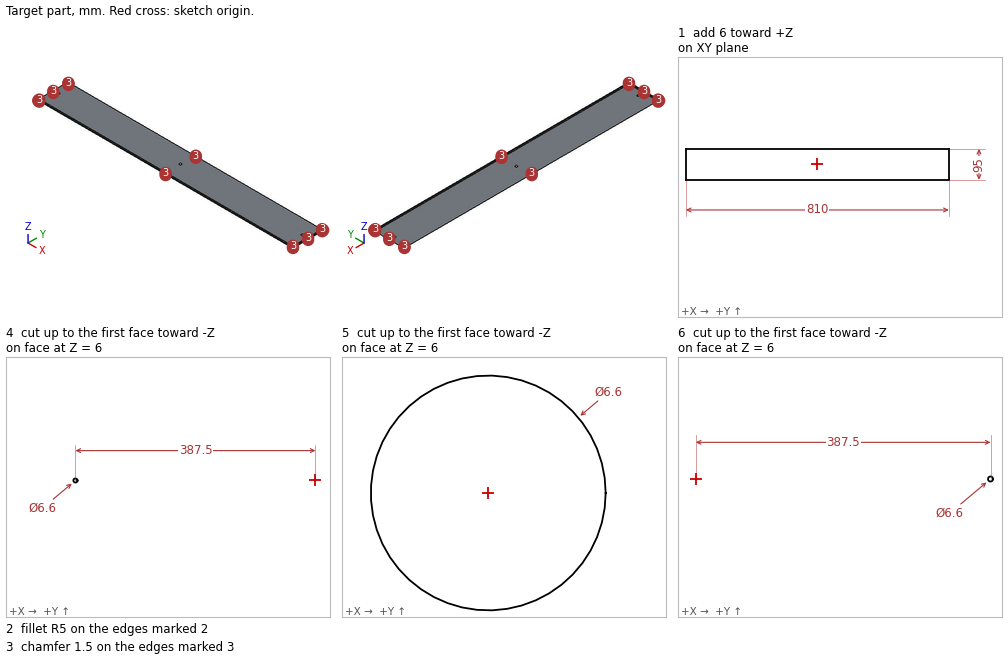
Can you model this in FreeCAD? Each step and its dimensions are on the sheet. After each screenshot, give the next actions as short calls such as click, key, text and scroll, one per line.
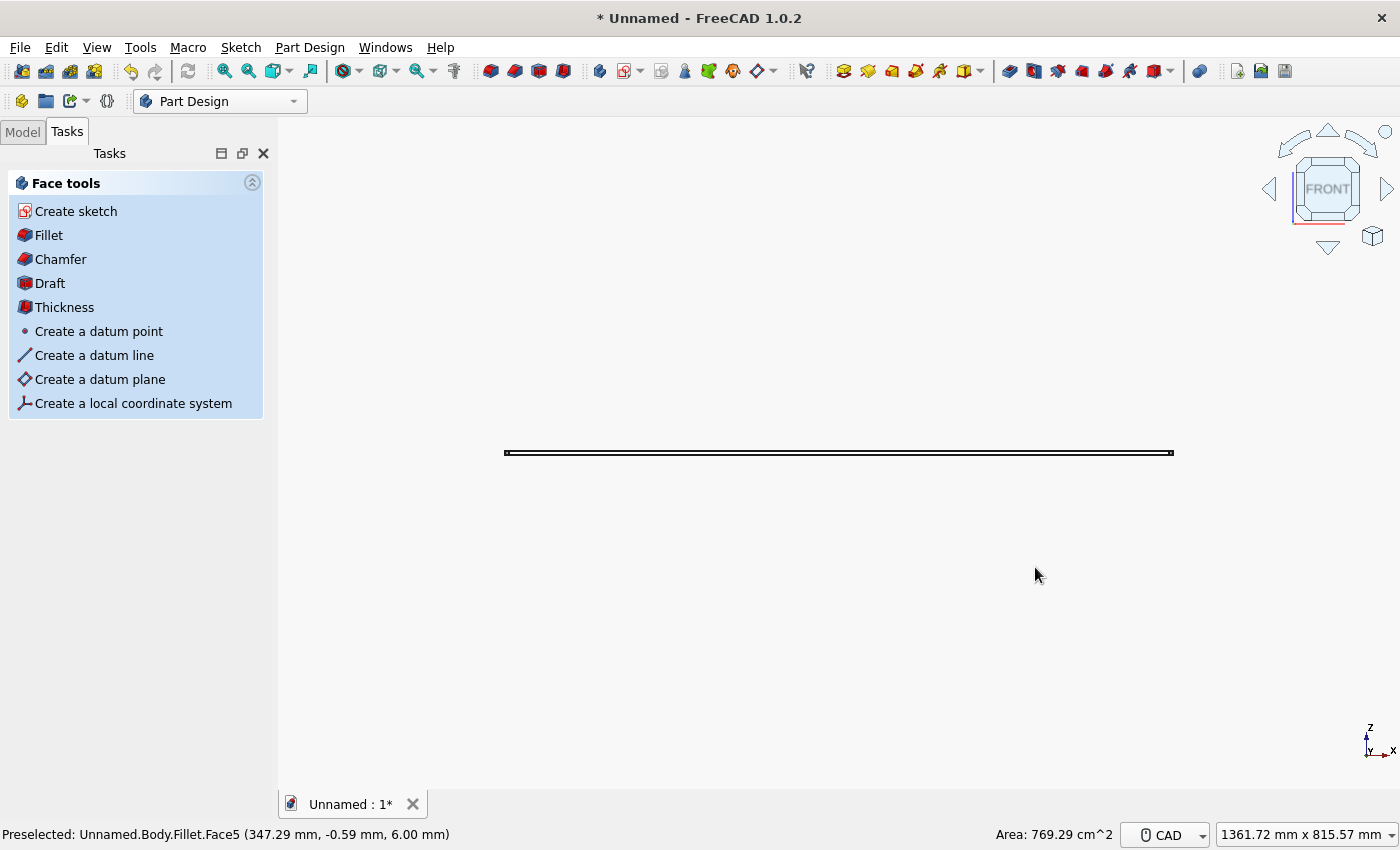
key(3)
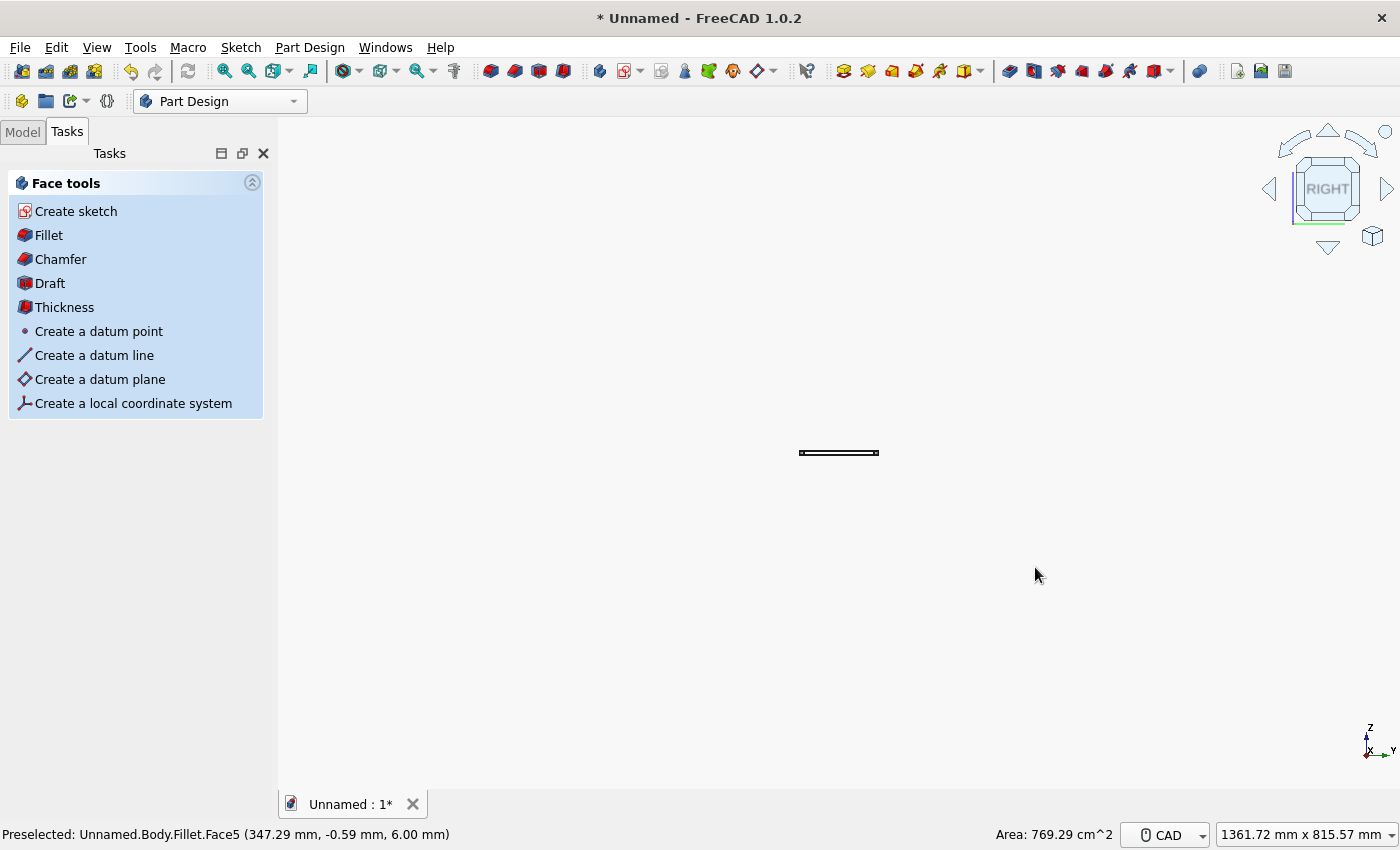
click(226, 72)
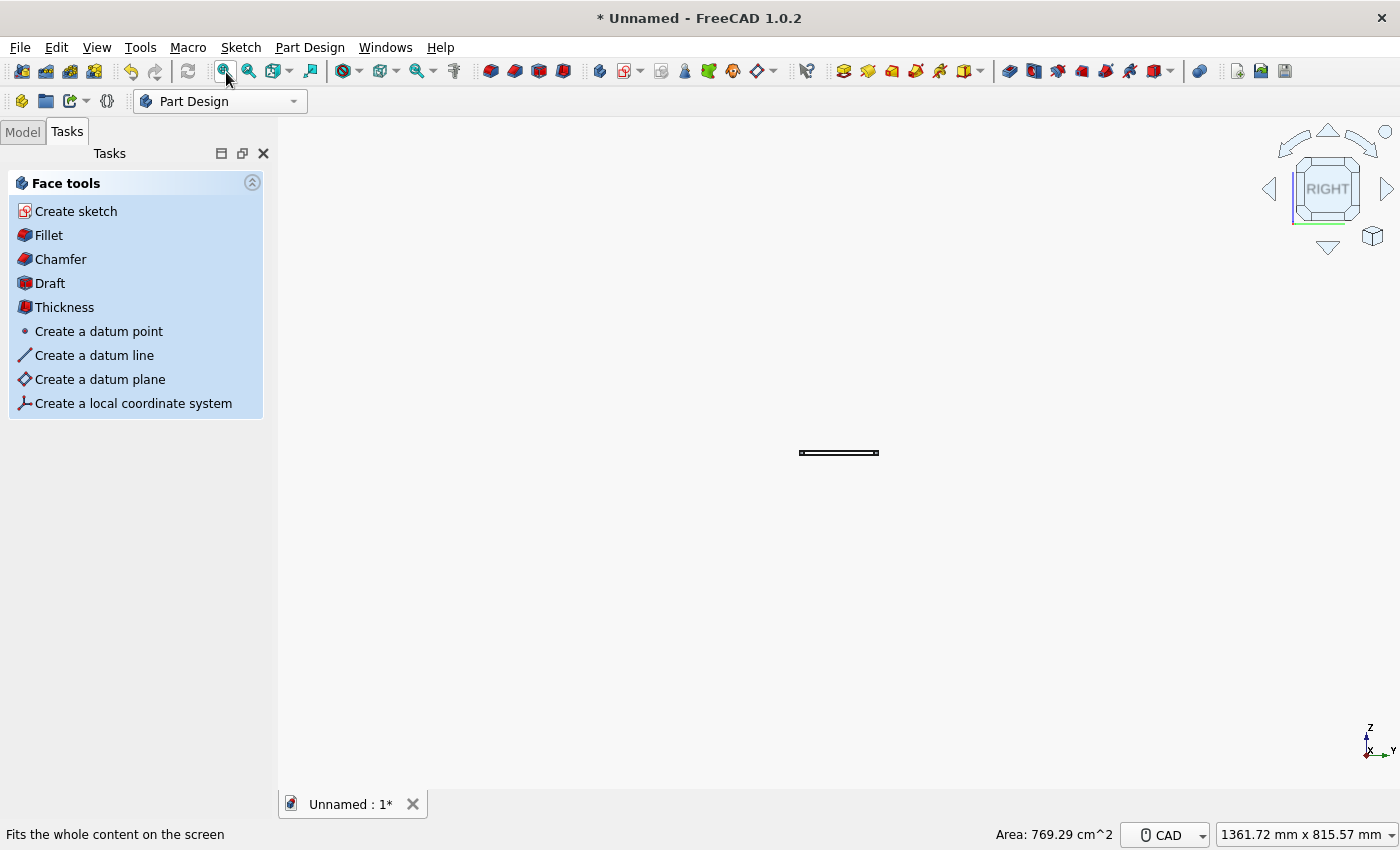
key(5)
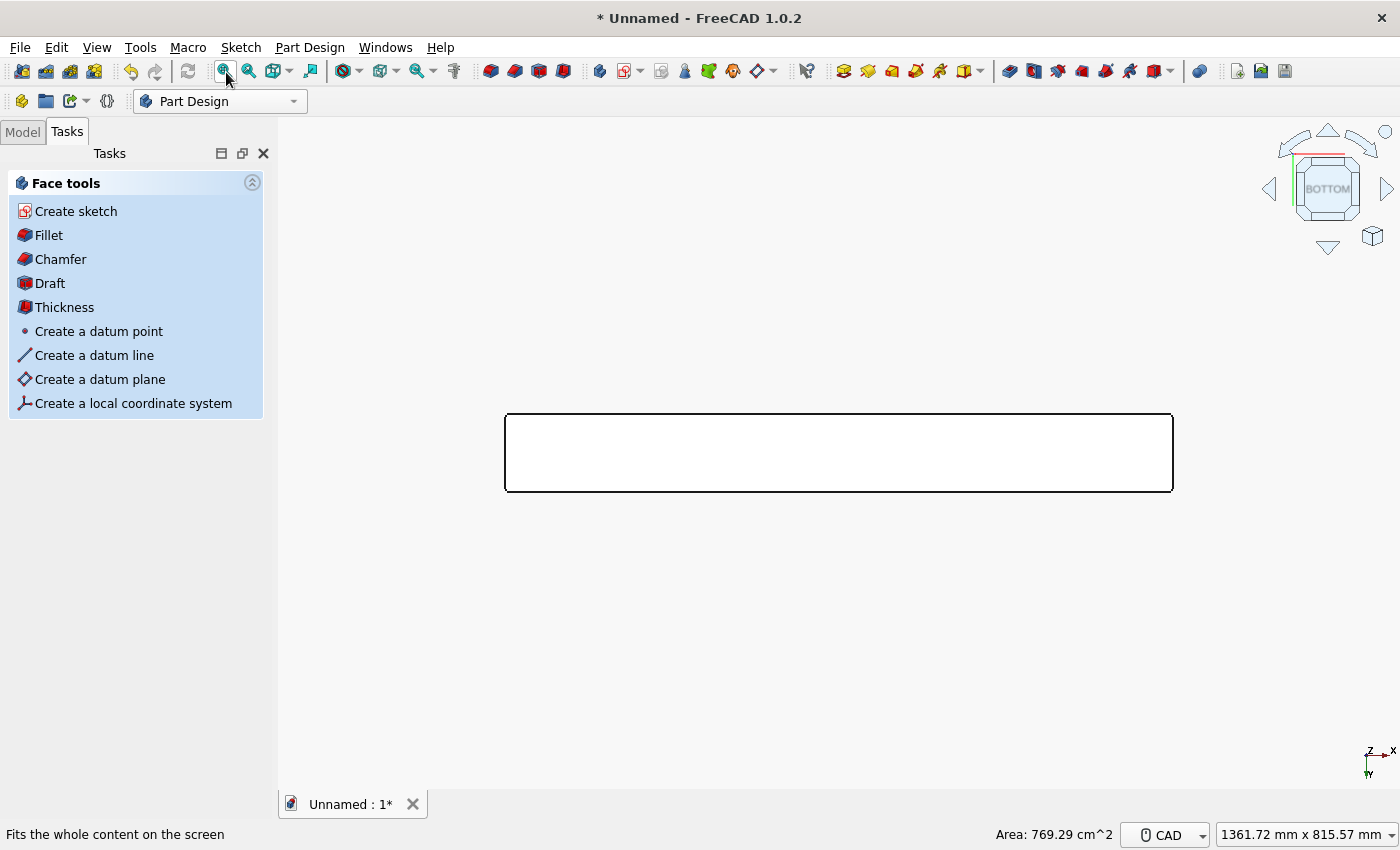
click(1125, 452, ctrl)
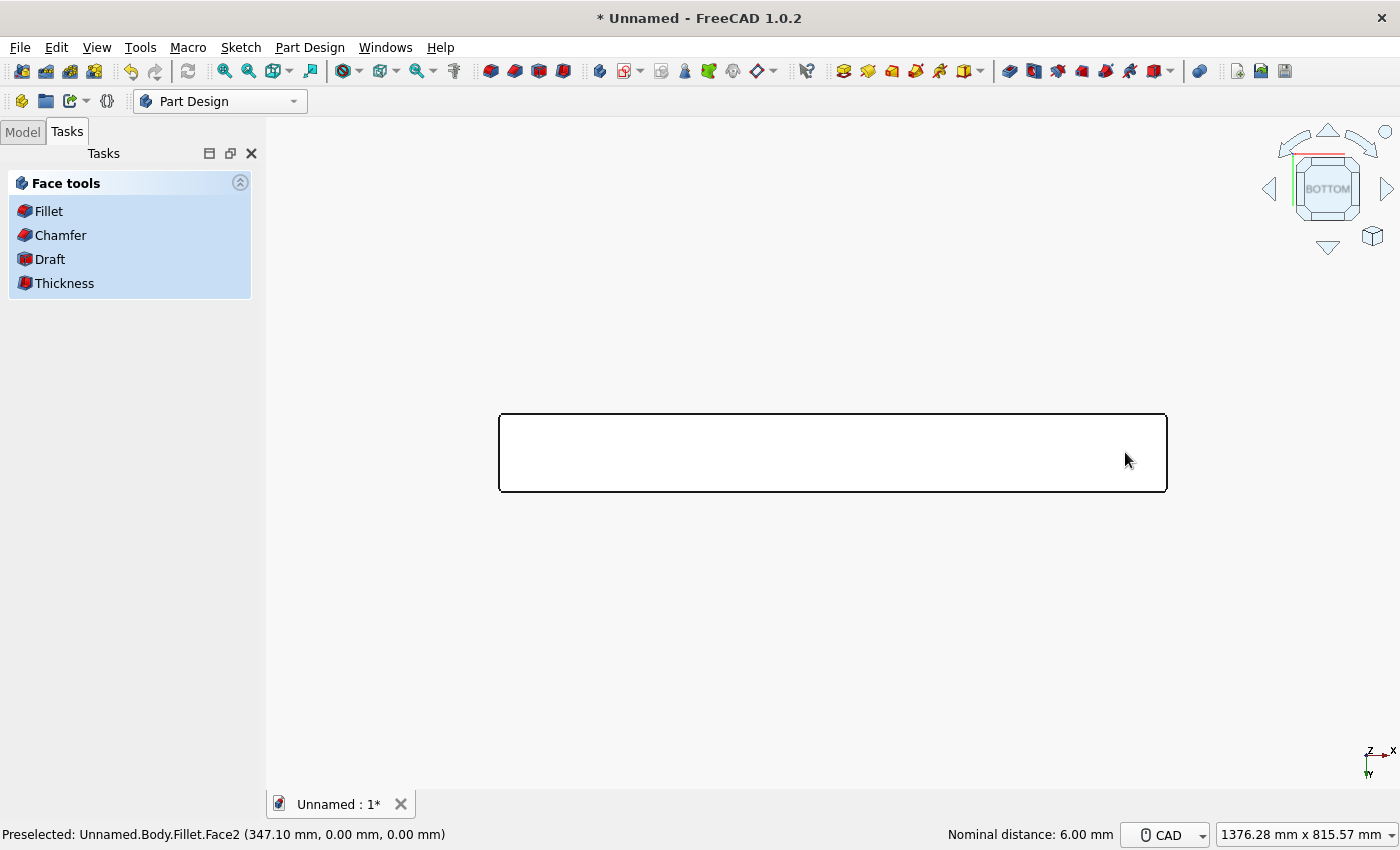
click(516, 72)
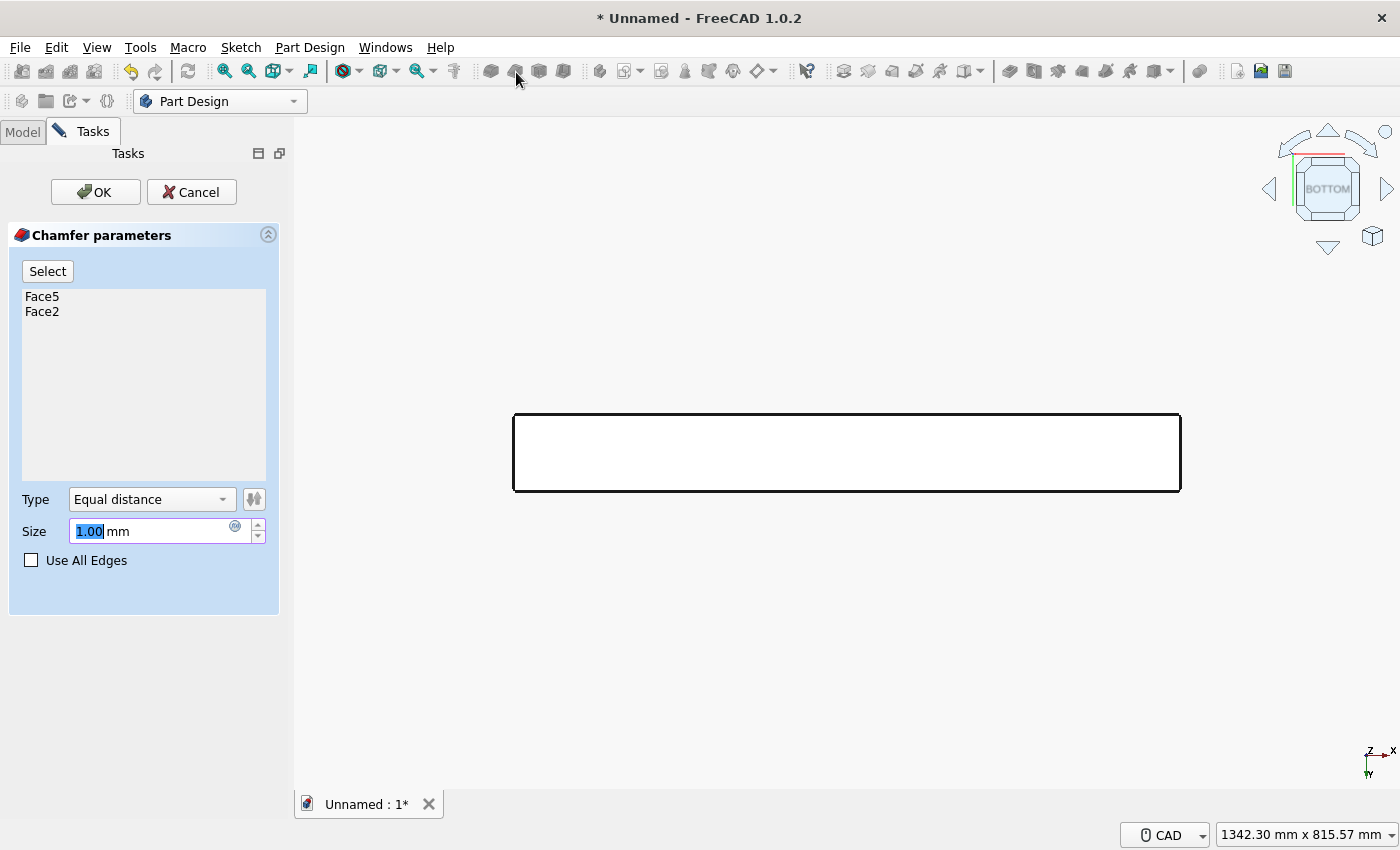
text(1.5)
key(Tab)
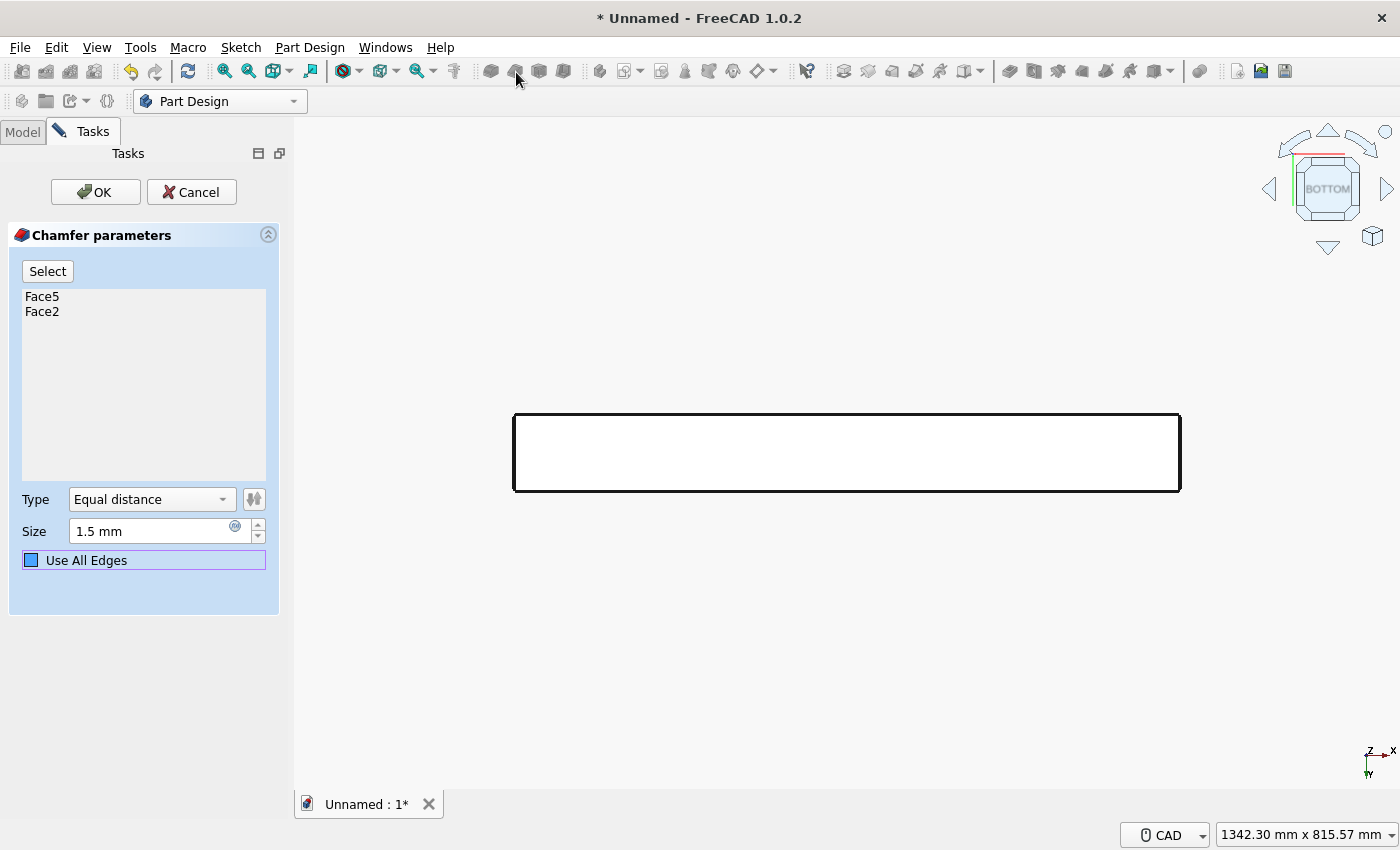
click(96, 192)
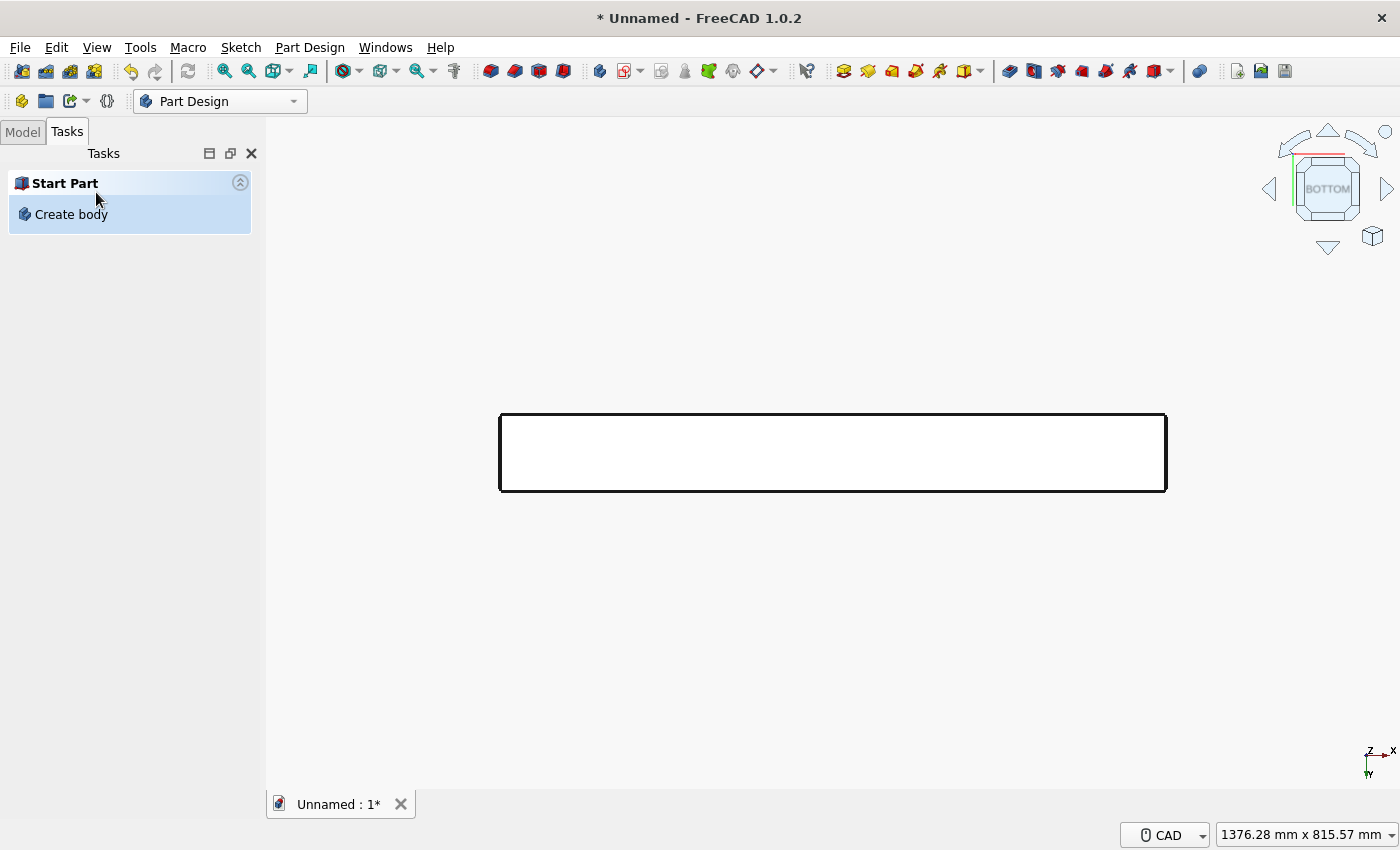
key(0)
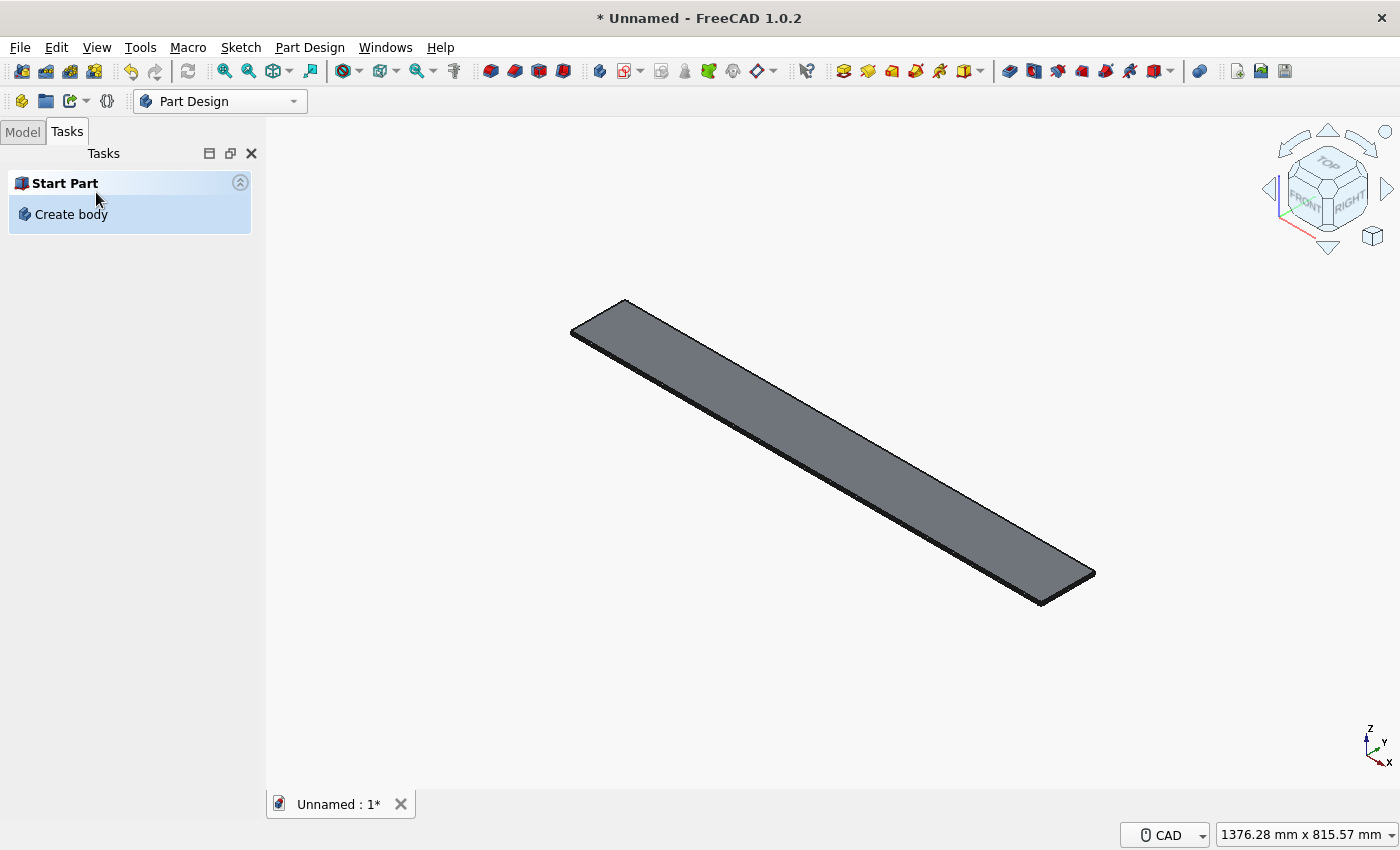
click(1035, 566)